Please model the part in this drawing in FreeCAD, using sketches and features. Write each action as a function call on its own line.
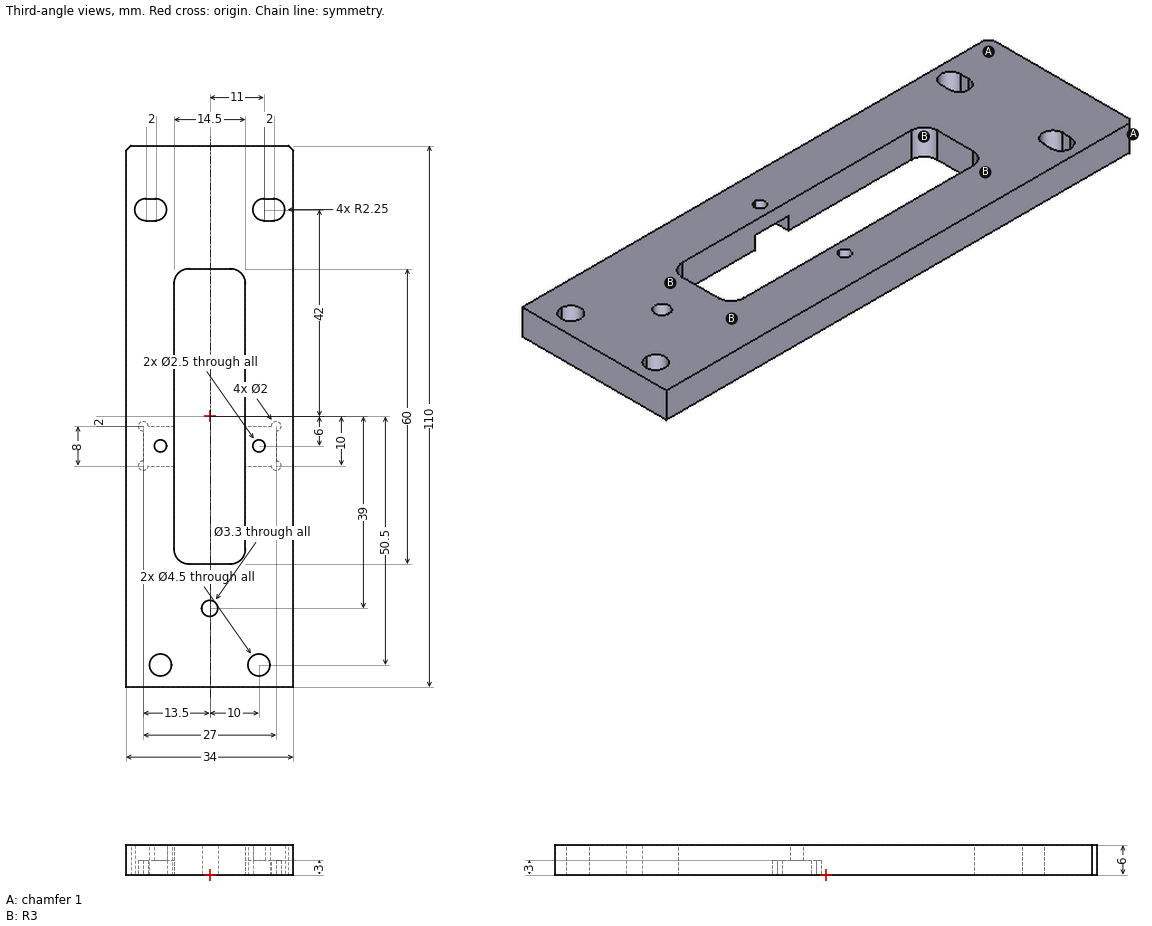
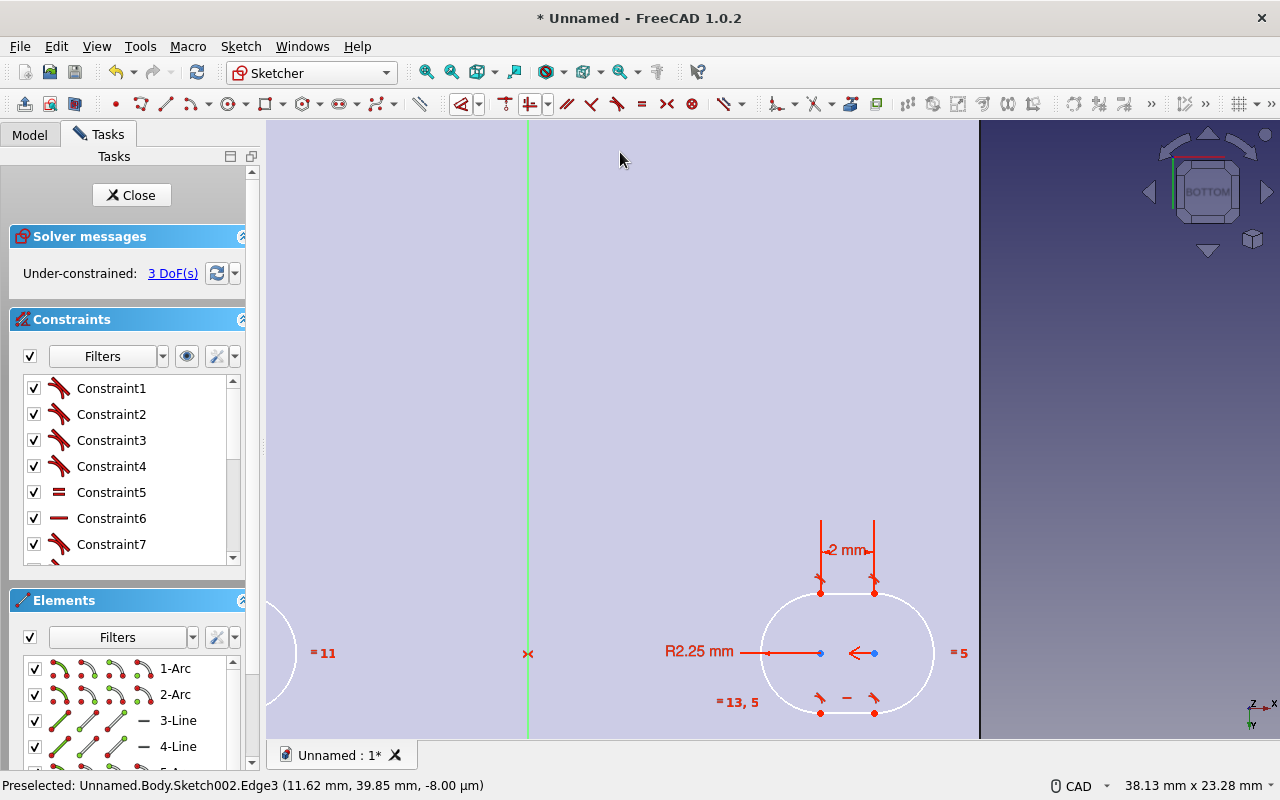
scroll(807, 608, down, 5)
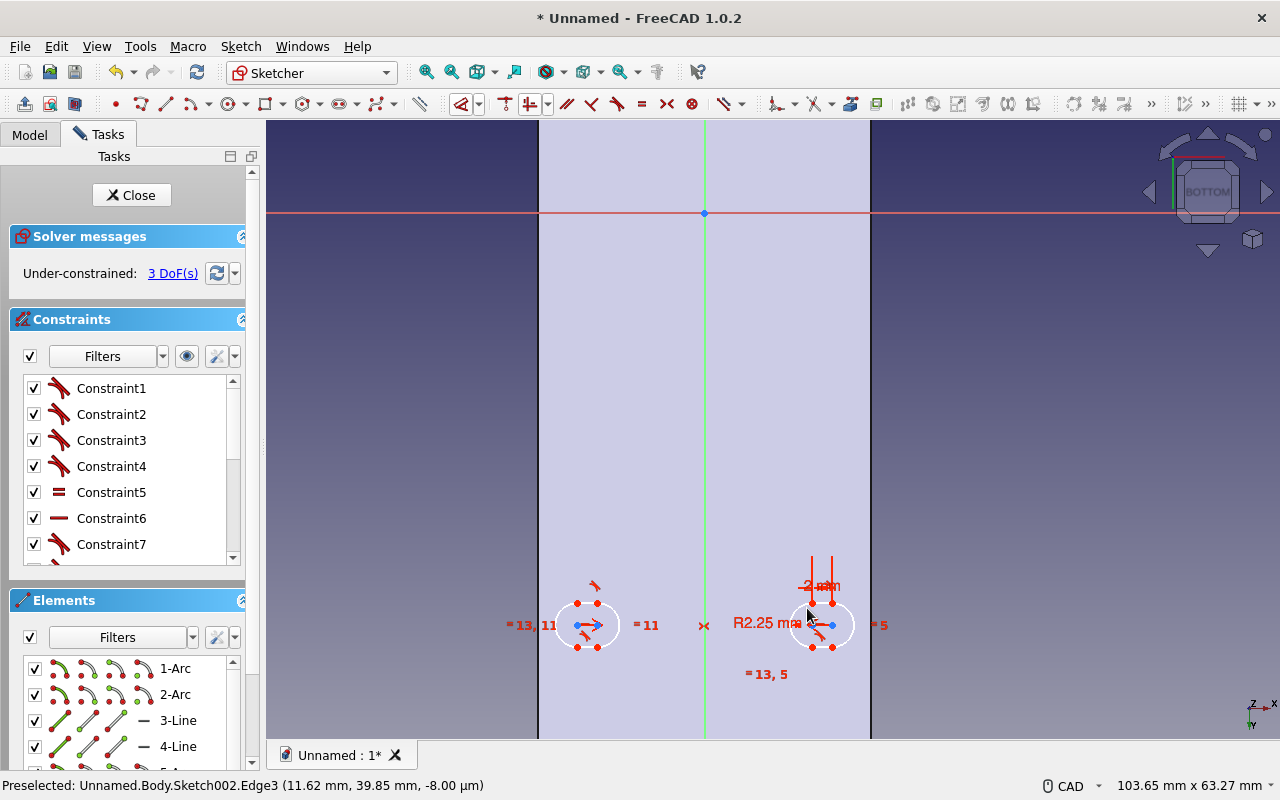
scroll(583, 603, up, 5)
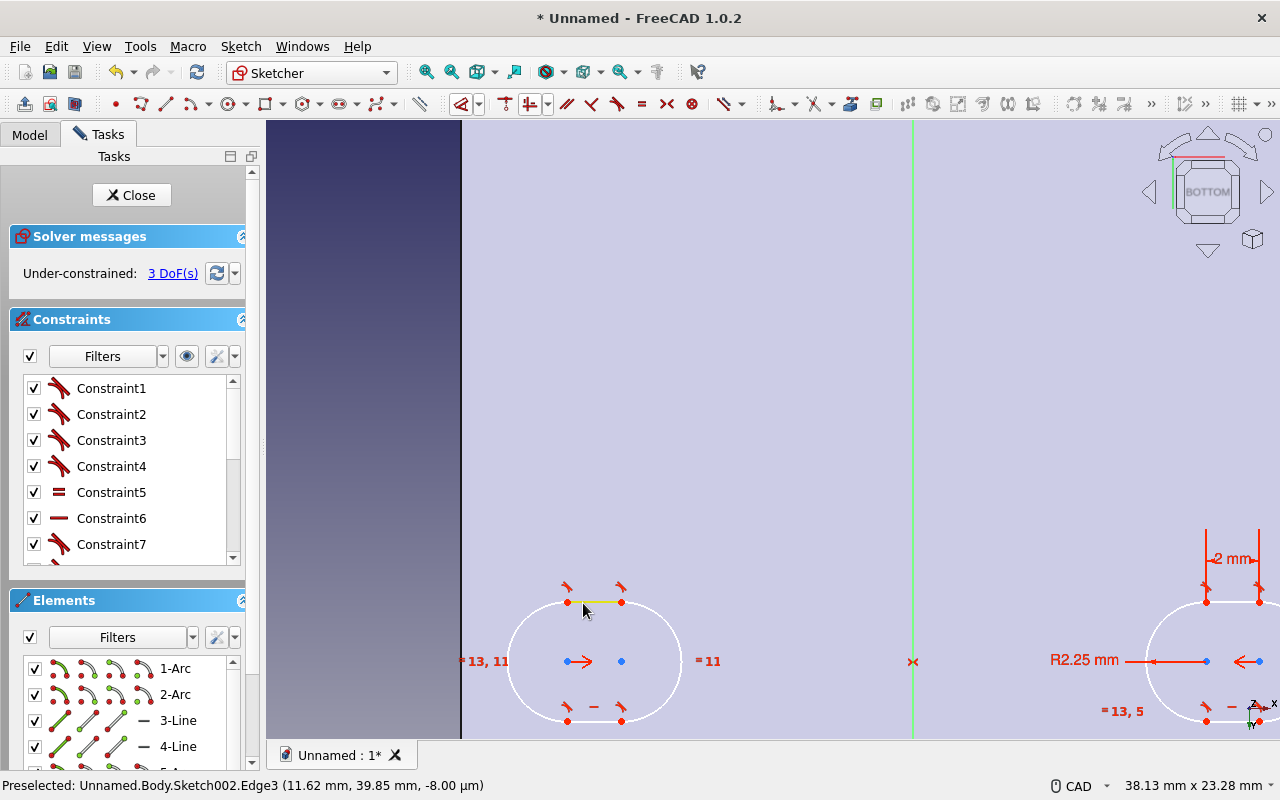
click(584, 602)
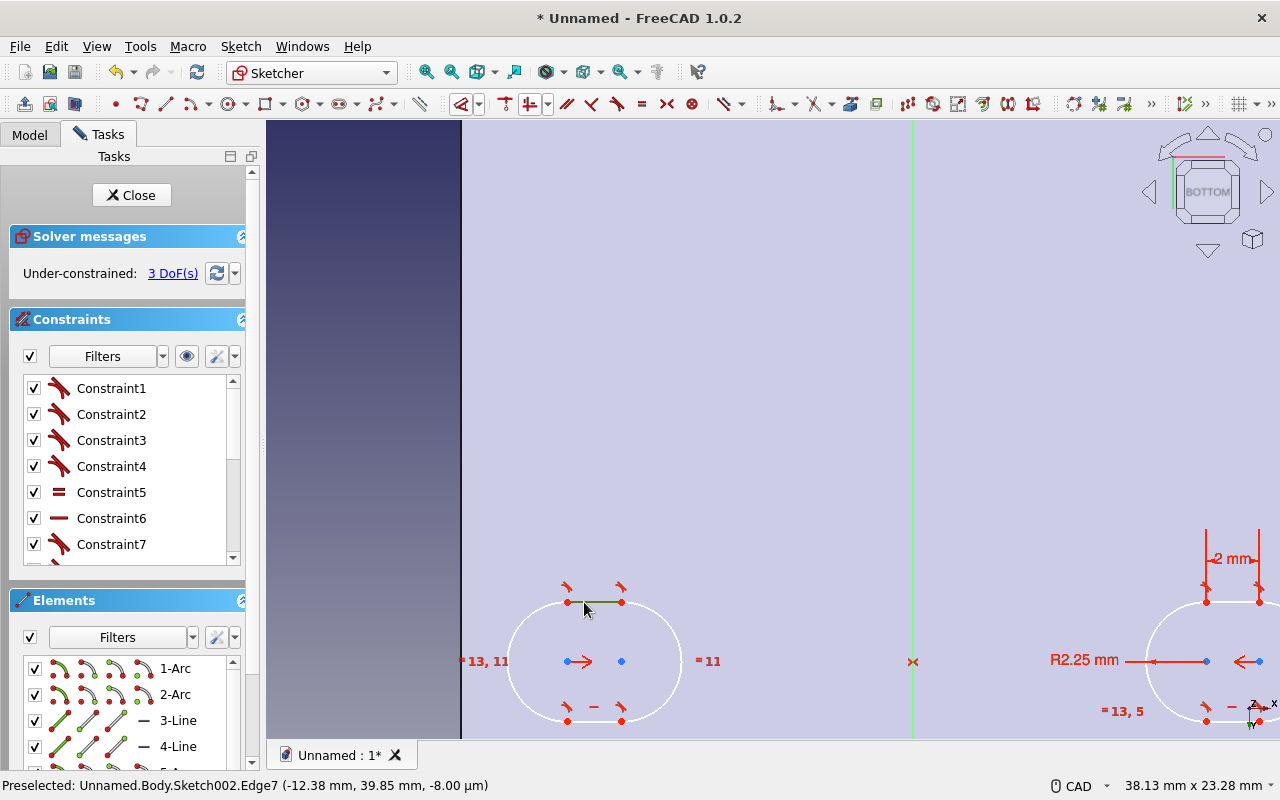
key(l)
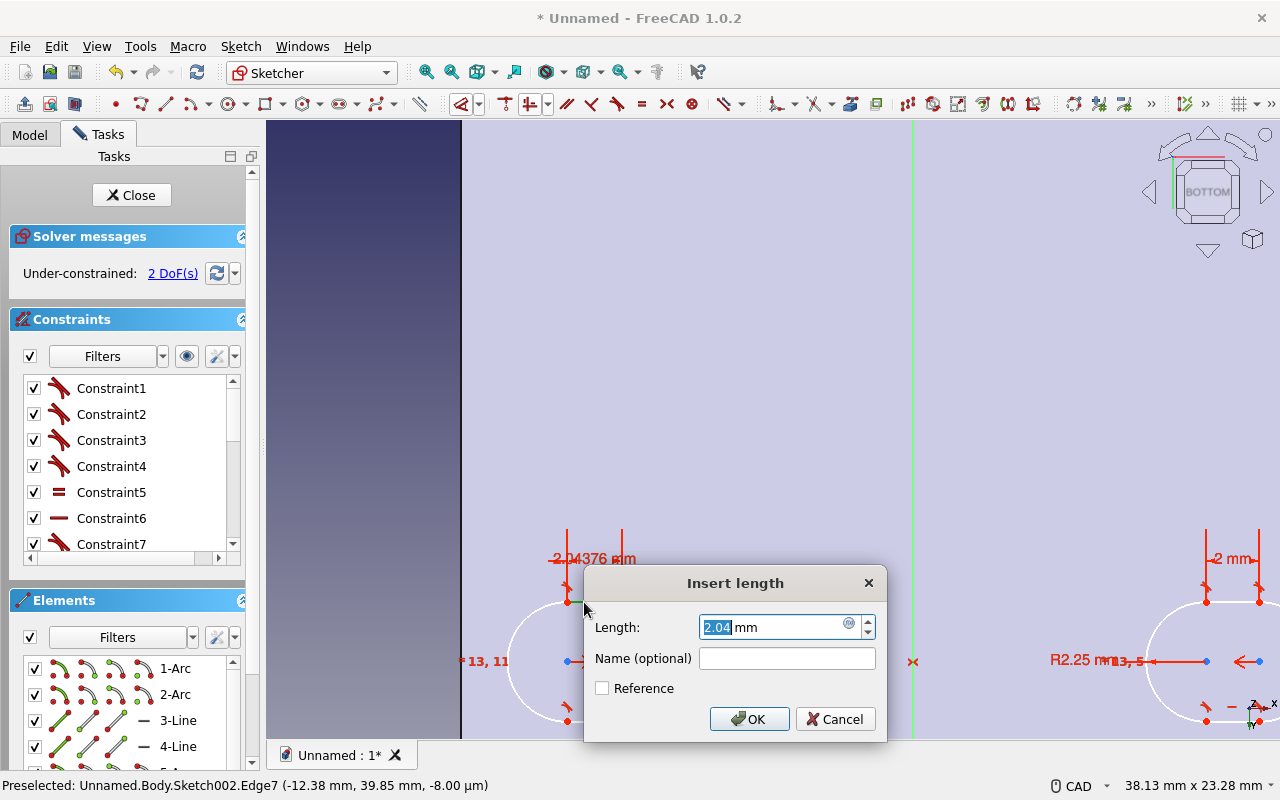
text(2)
key(Return)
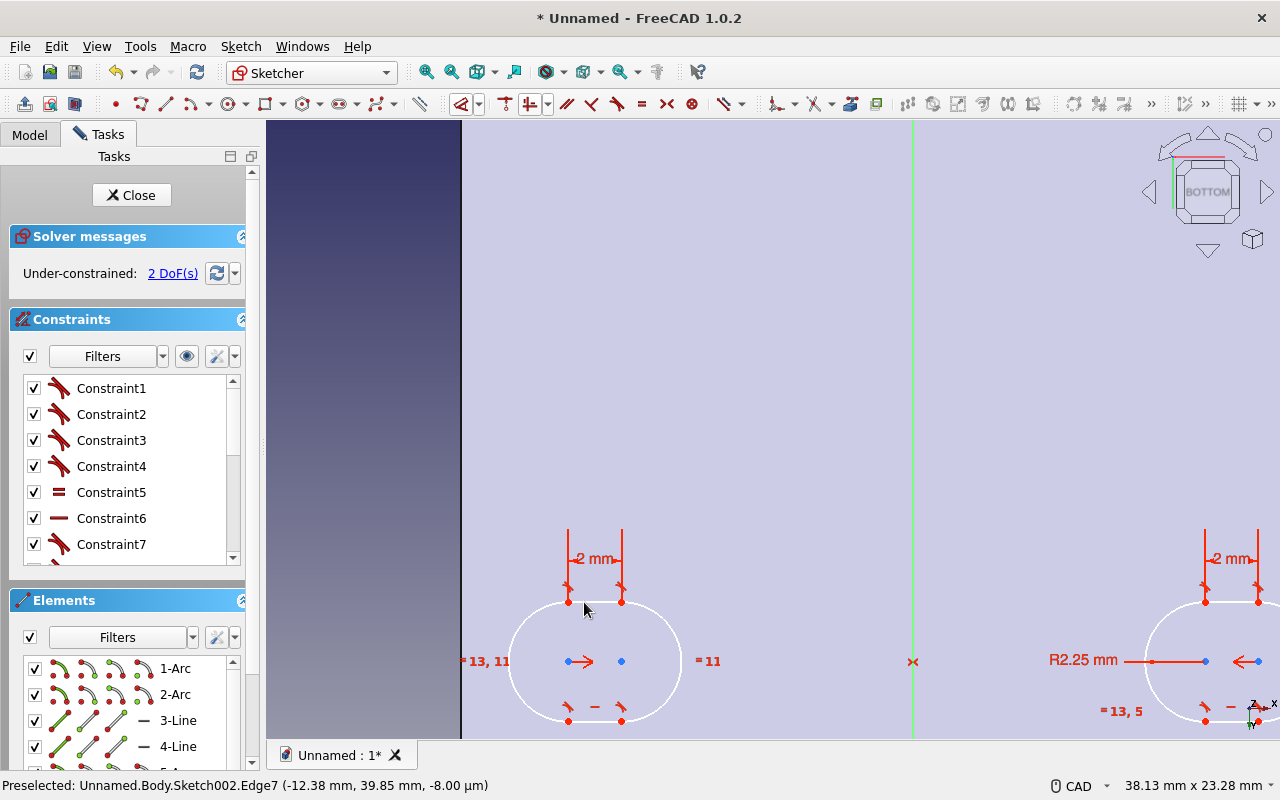
scroll(583, 603, down, 5)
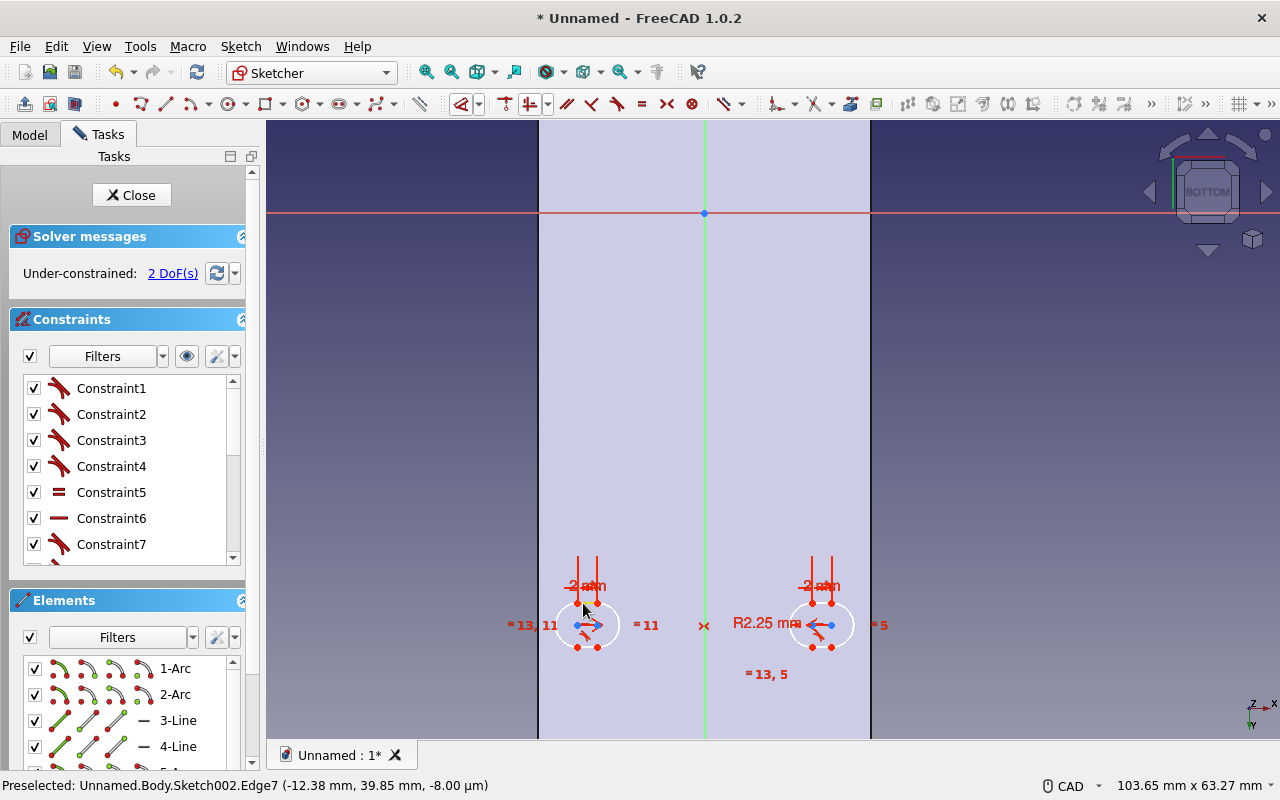
click(812, 603)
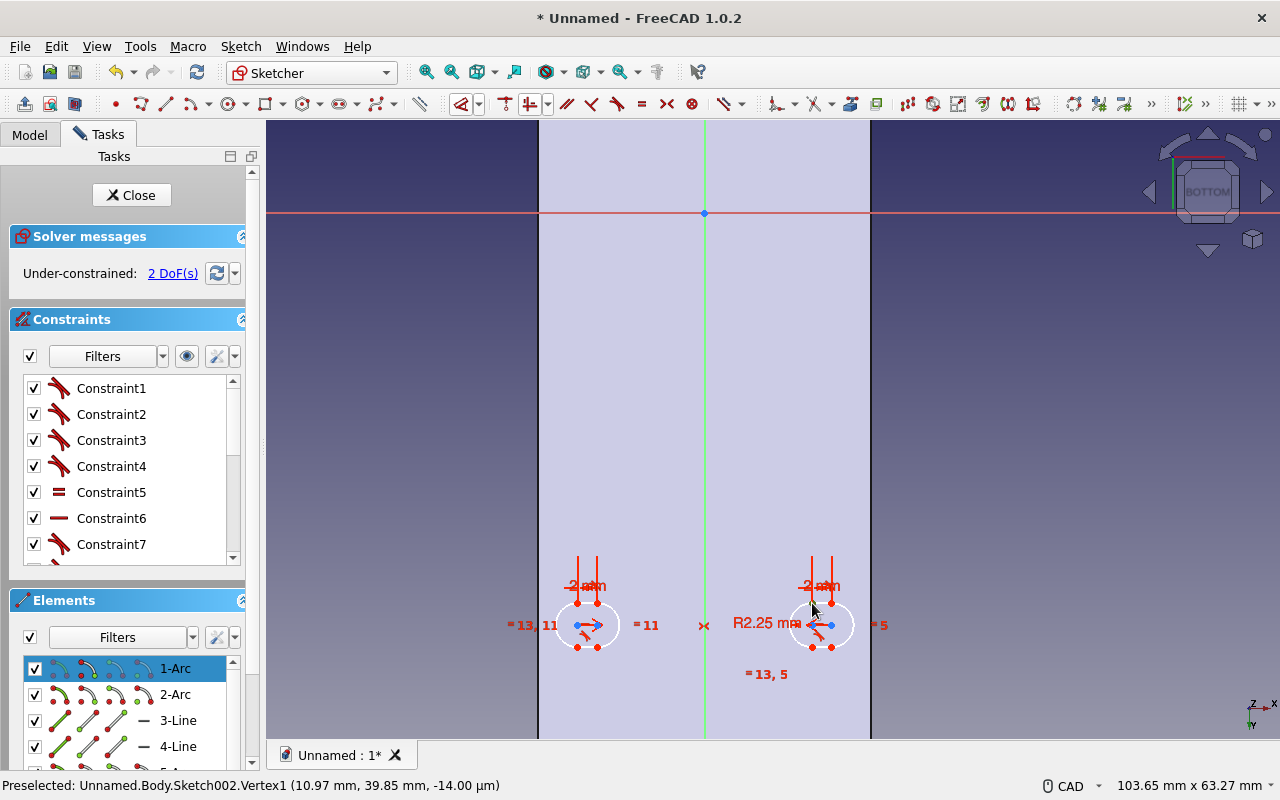
key(l)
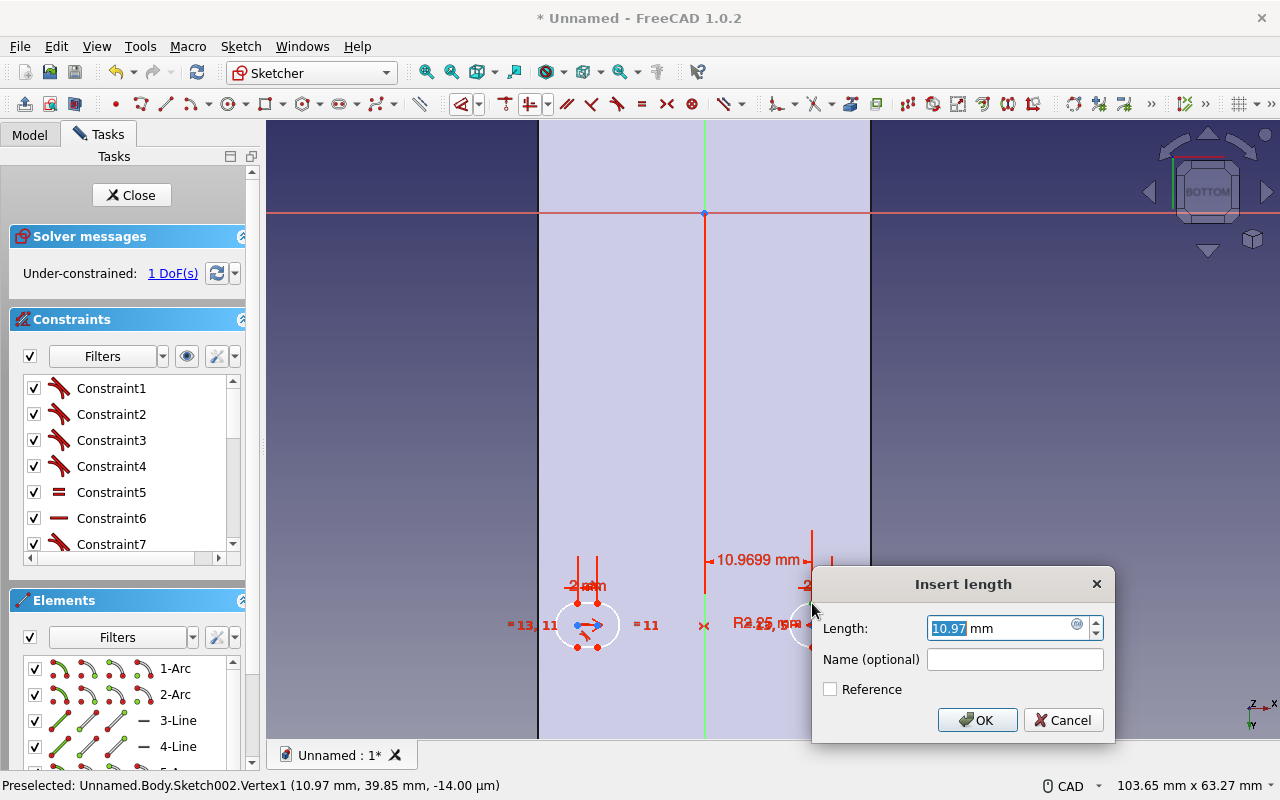
text(11)
key(Return)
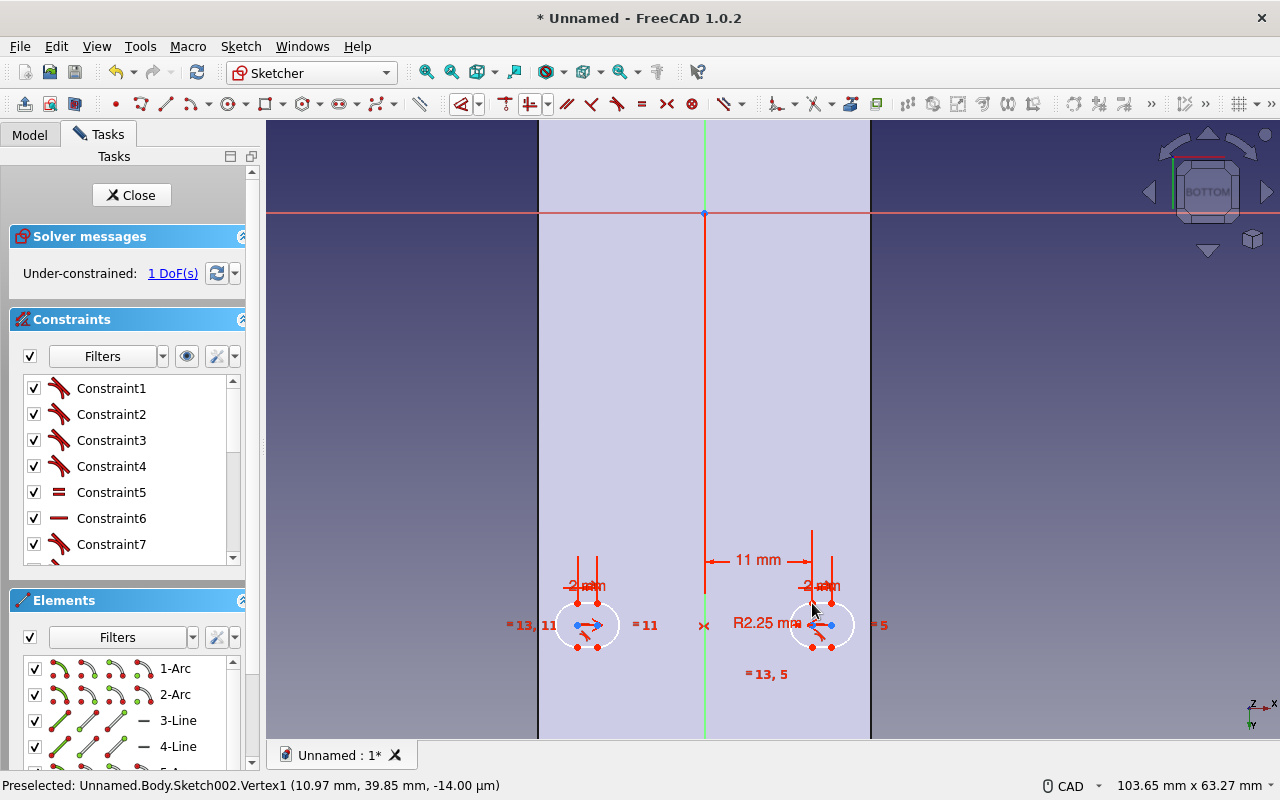
click(812, 625)